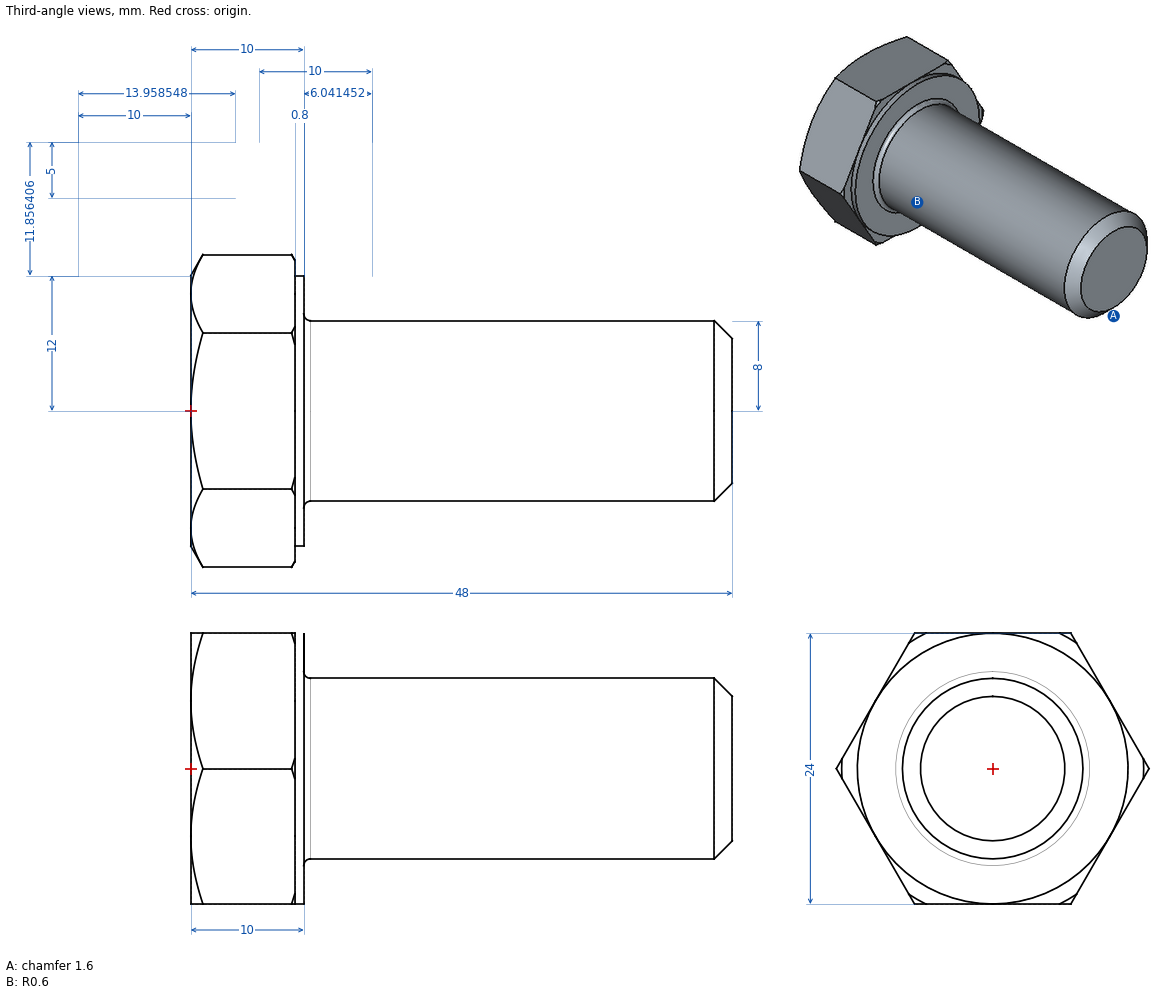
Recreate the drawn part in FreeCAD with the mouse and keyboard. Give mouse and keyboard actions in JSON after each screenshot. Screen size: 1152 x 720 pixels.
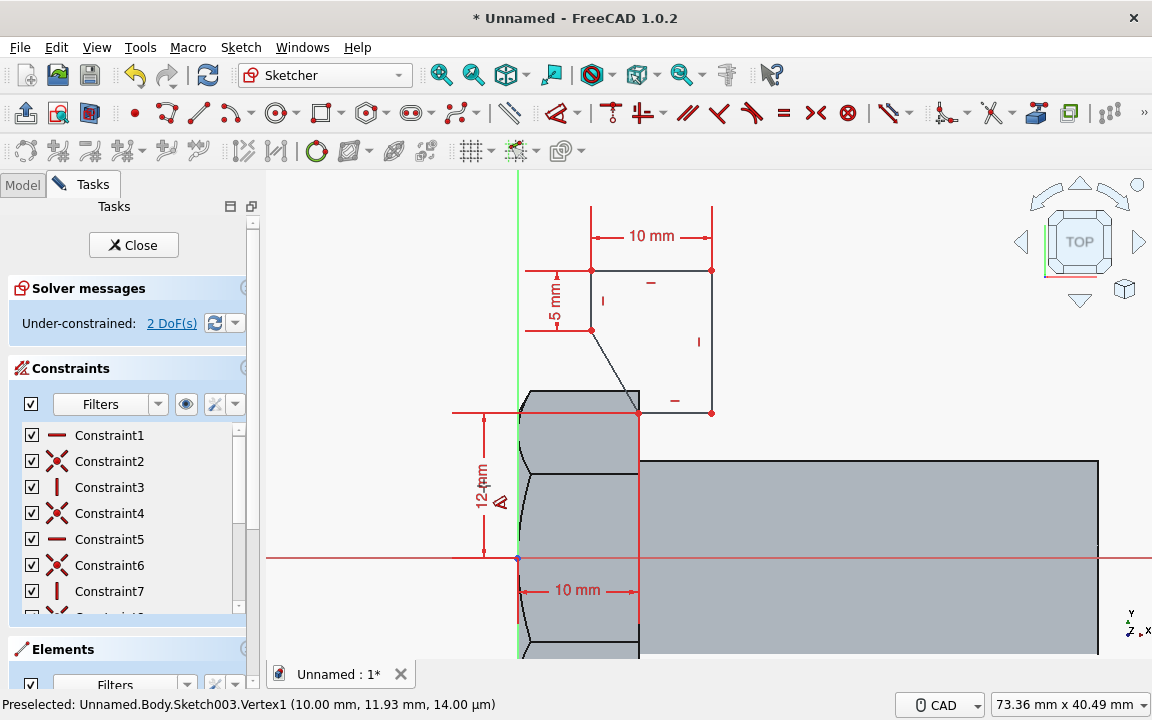
{"action": "left_click", "coordinate": [661, 413]}
{"action": "left_click", "coordinate": [675, 379]}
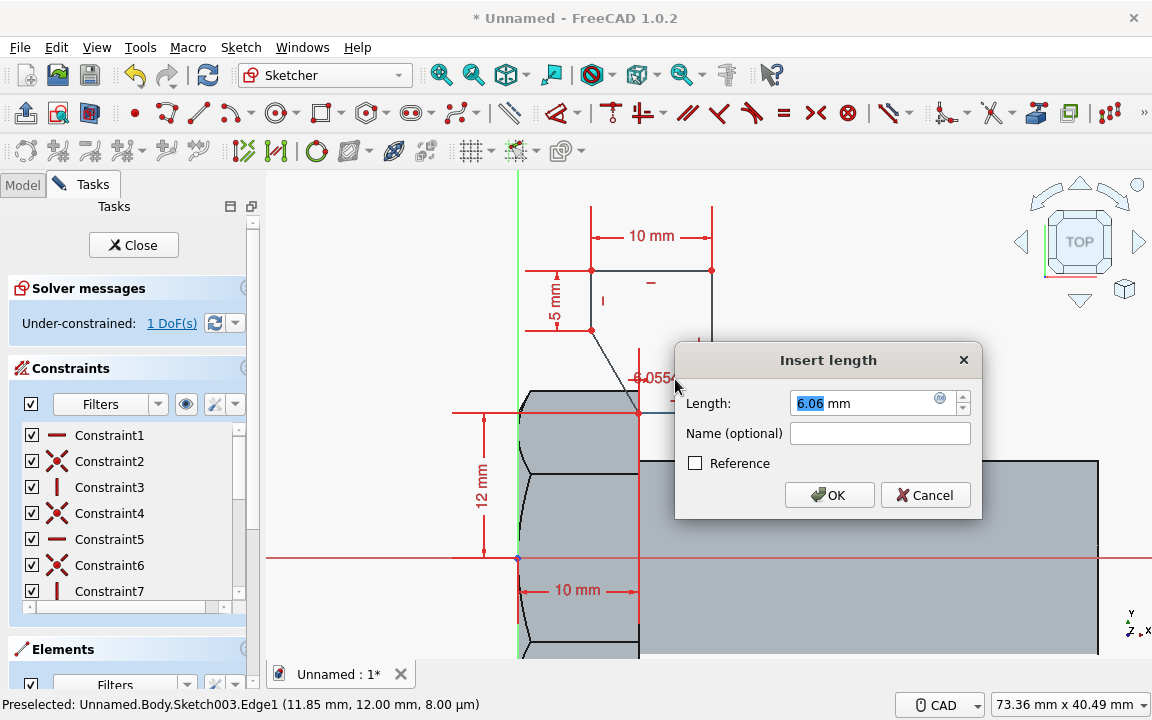
{"action": "type", "text": "6.041452"}
{"action": "key", "text": "Return"}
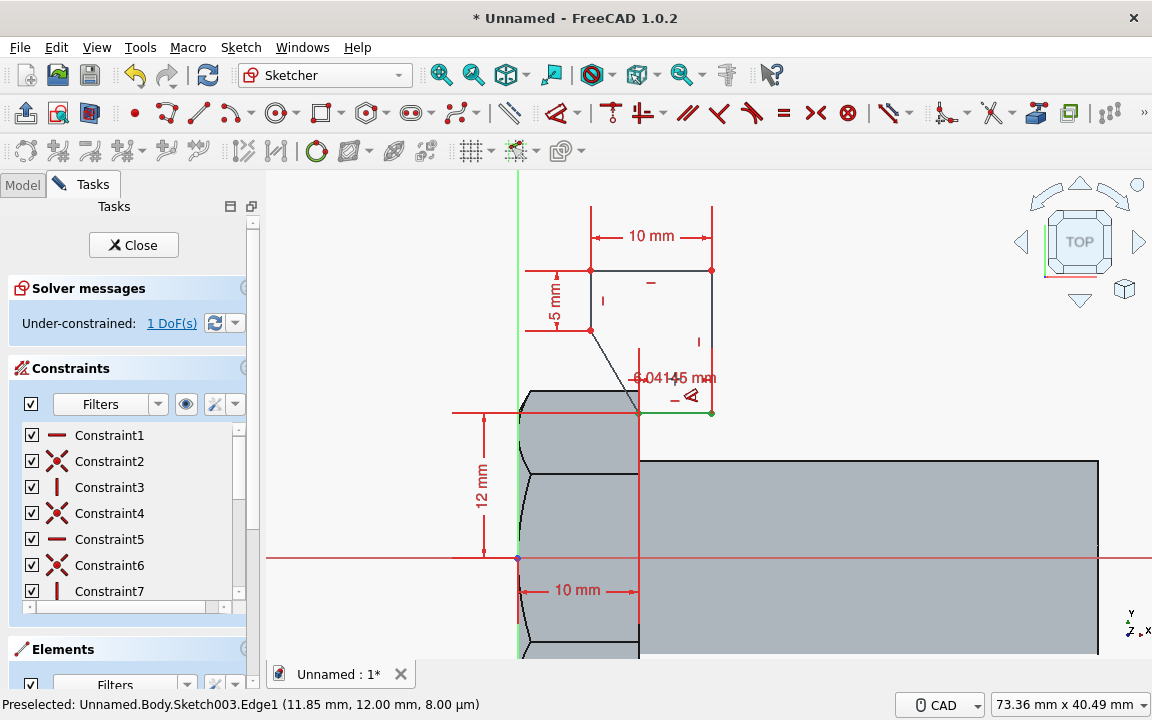
{"action": "left_click", "coordinate": [712, 370]}
{"action": "left_click", "coordinate": [746, 342]}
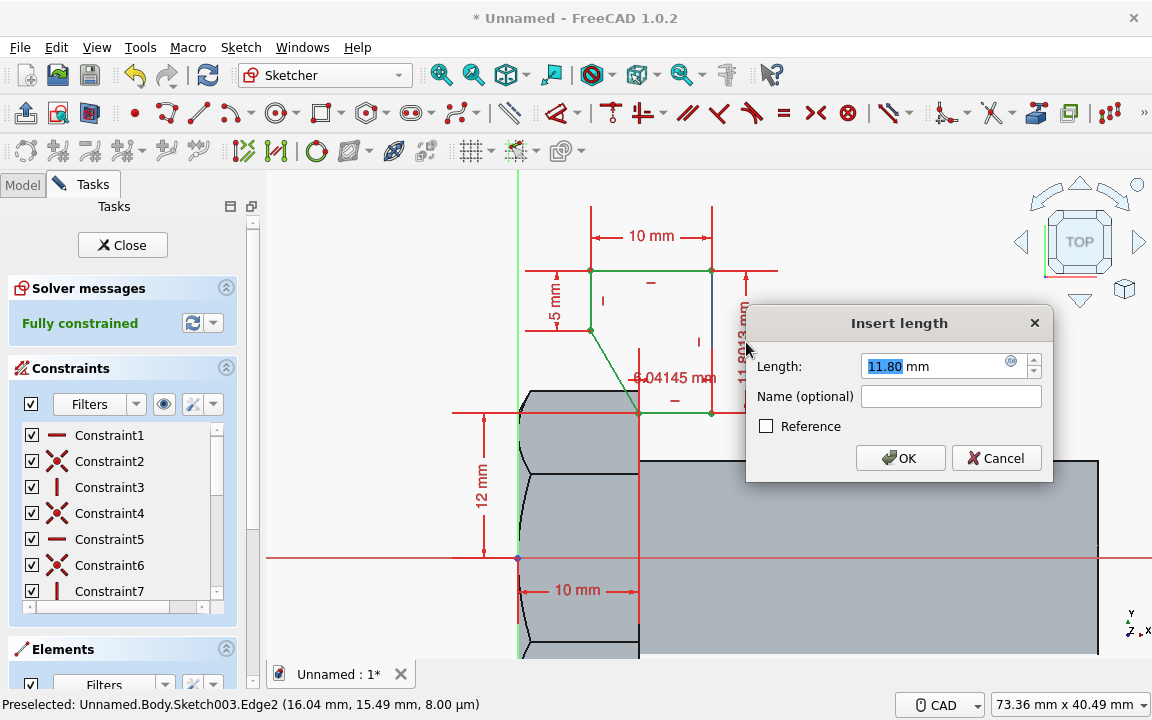
{"action": "type", "text": "11.856406"}
{"action": "key", "text": "Return"}
{"action": "key", "text": "Escape"}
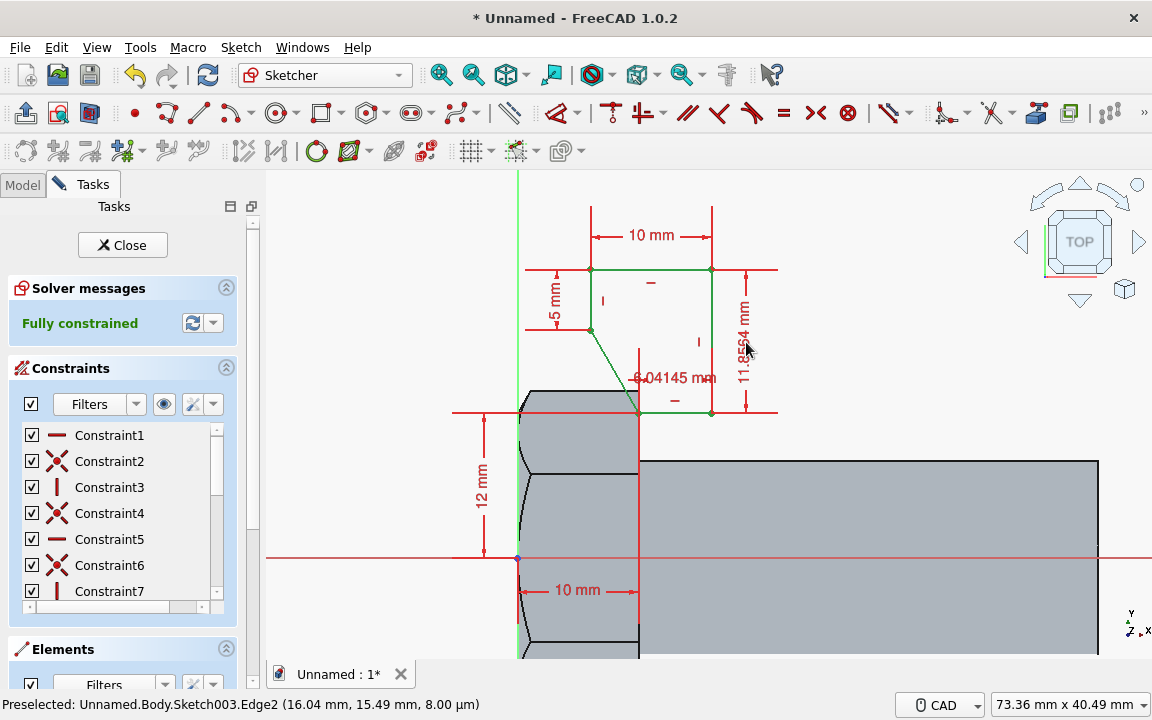
{"action": "left_click", "coordinate": [123, 245]}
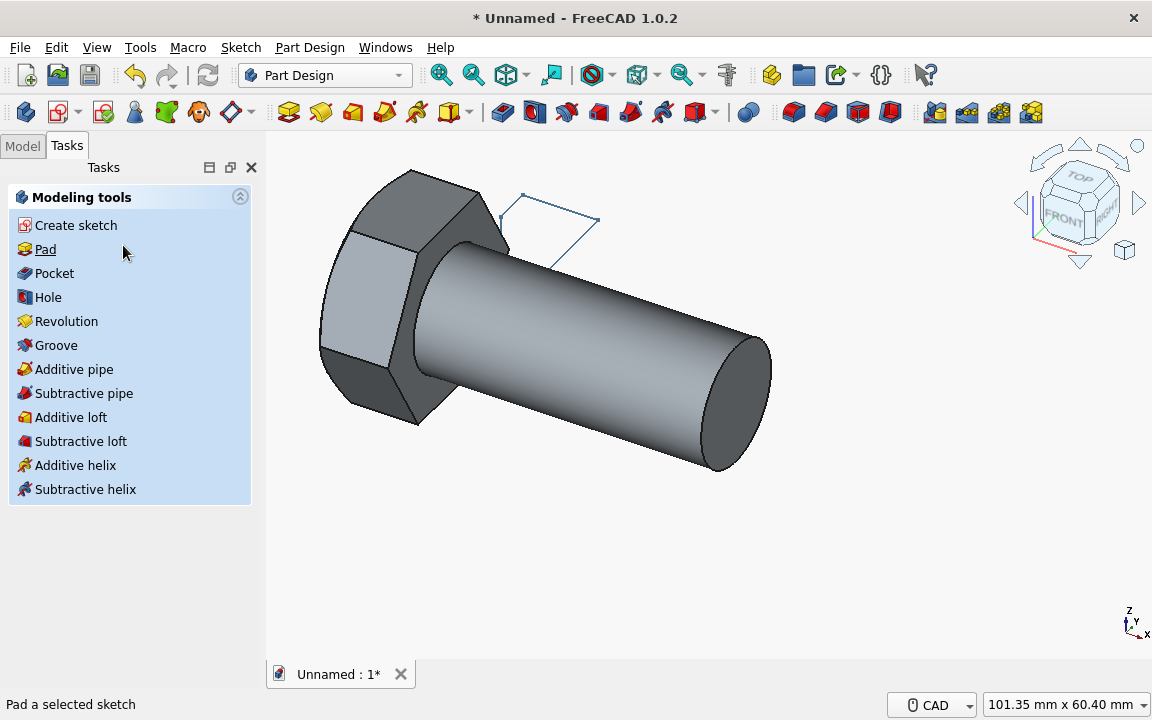
{"action": "left_click", "coordinate": [568, 112]}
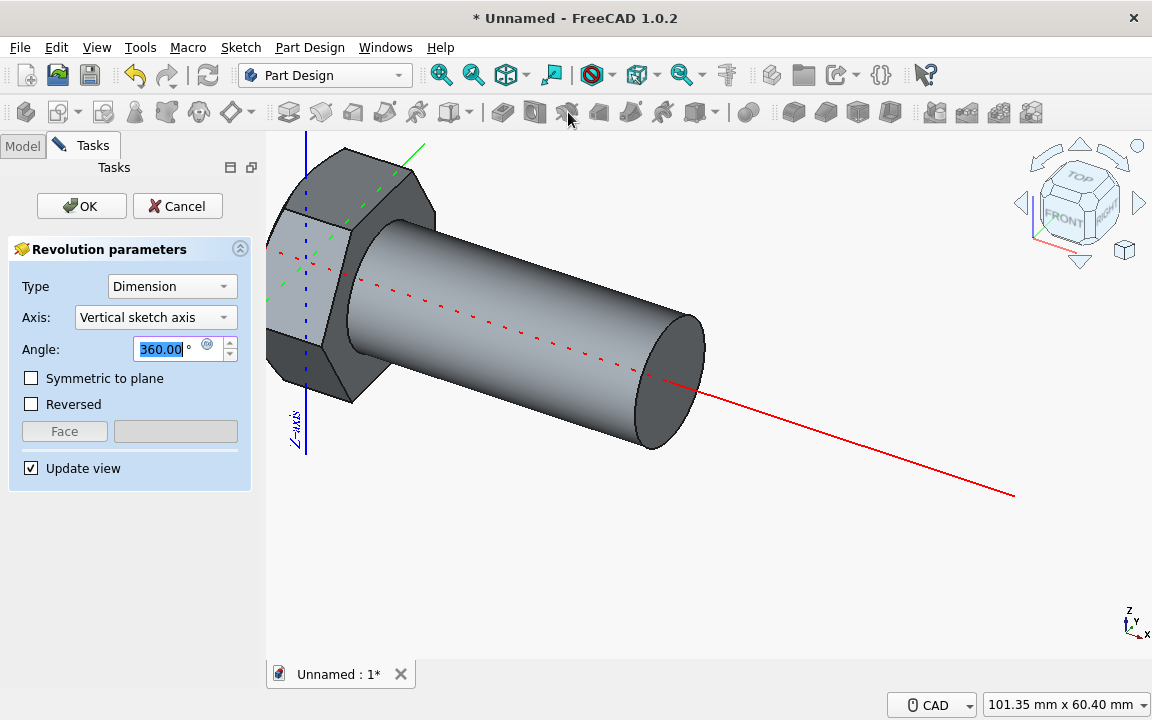
{"action": "left_click", "coordinate": [156, 318]}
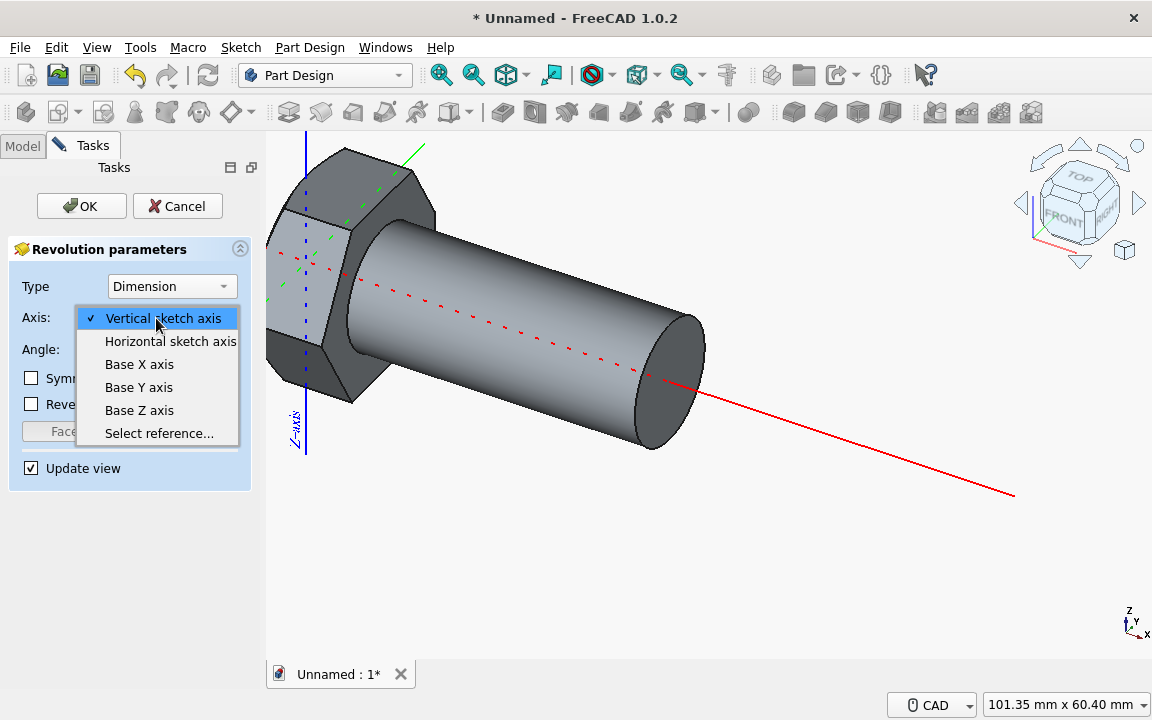
{"action": "left_click", "coordinate": [156, 342]}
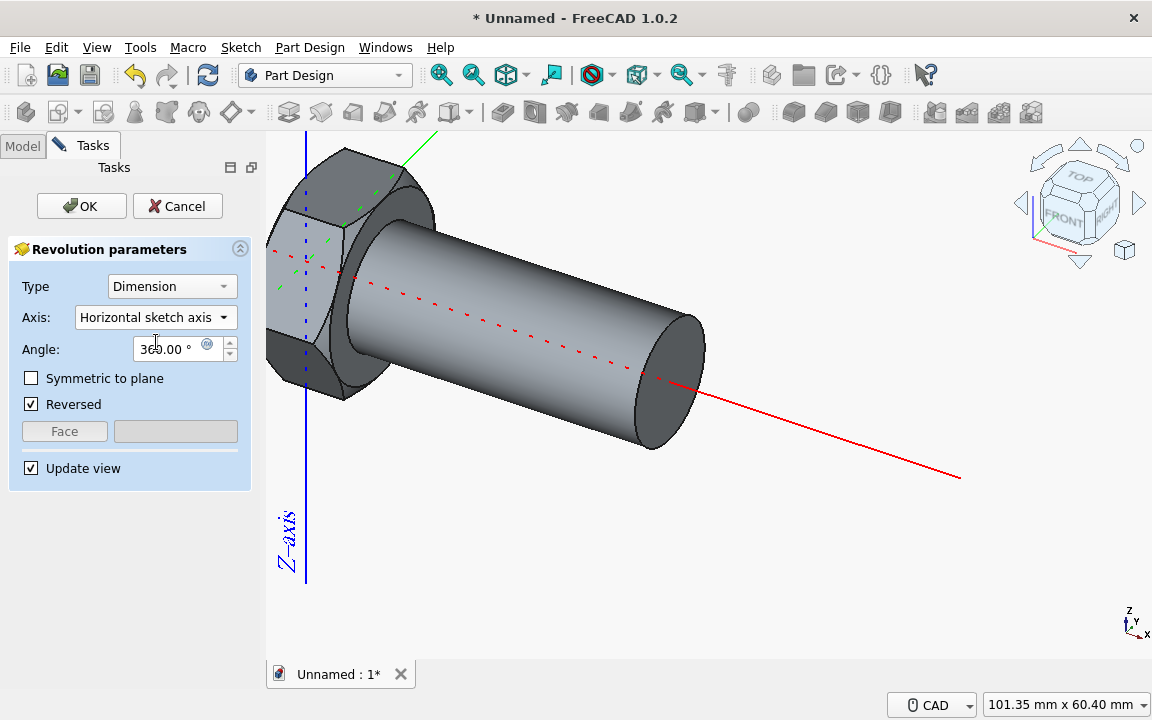
{"action": "left_click", "coordinate": [82, 206]}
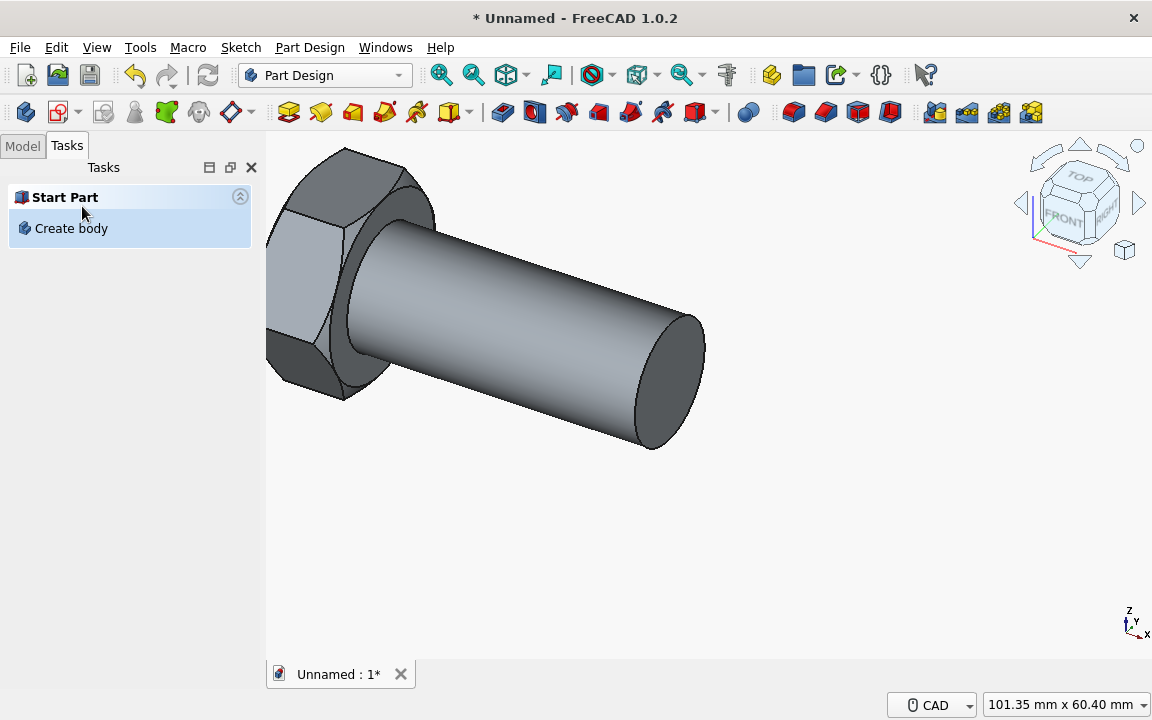
{"action": "left_click", "coordinate": [442, 76]}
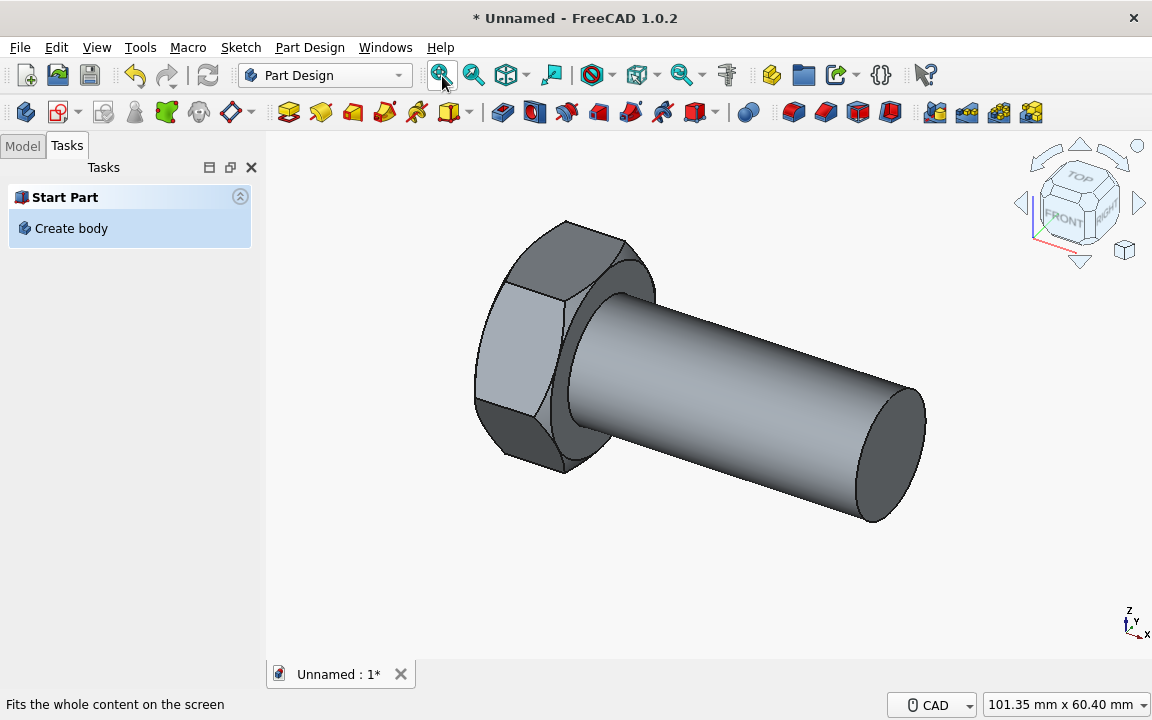
{"action": "left_click", "coordinate": [58, 112]}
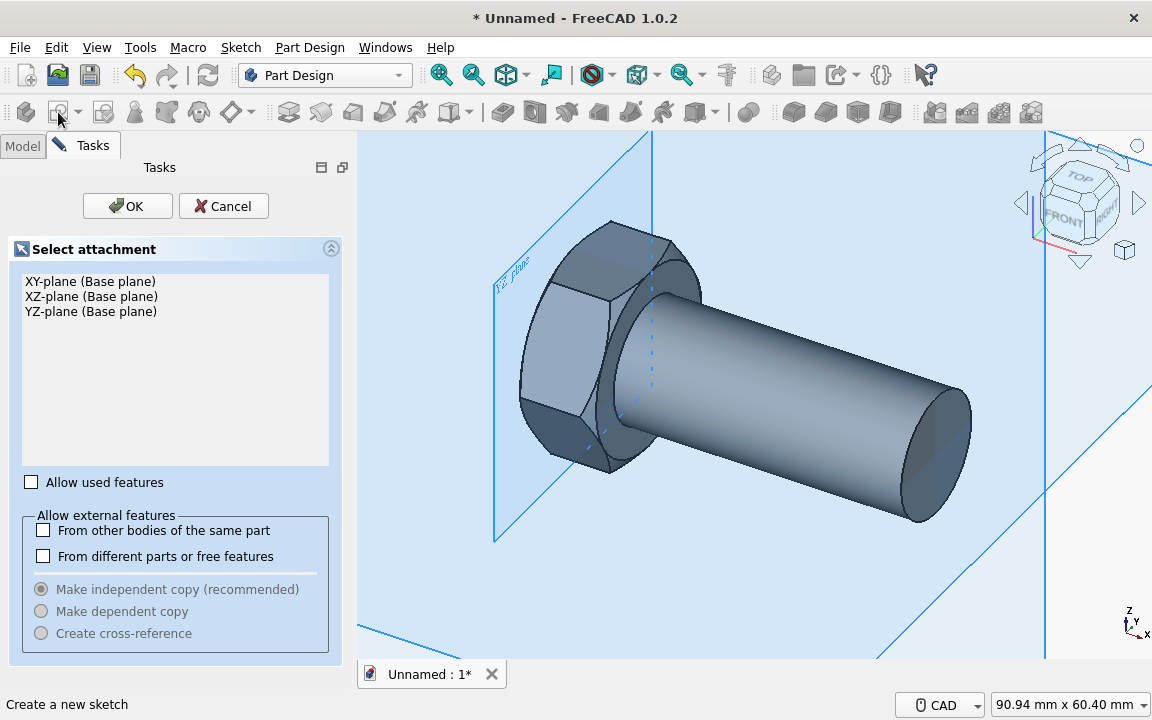
{"action": "left_click", "coordinate": [82, 282]}